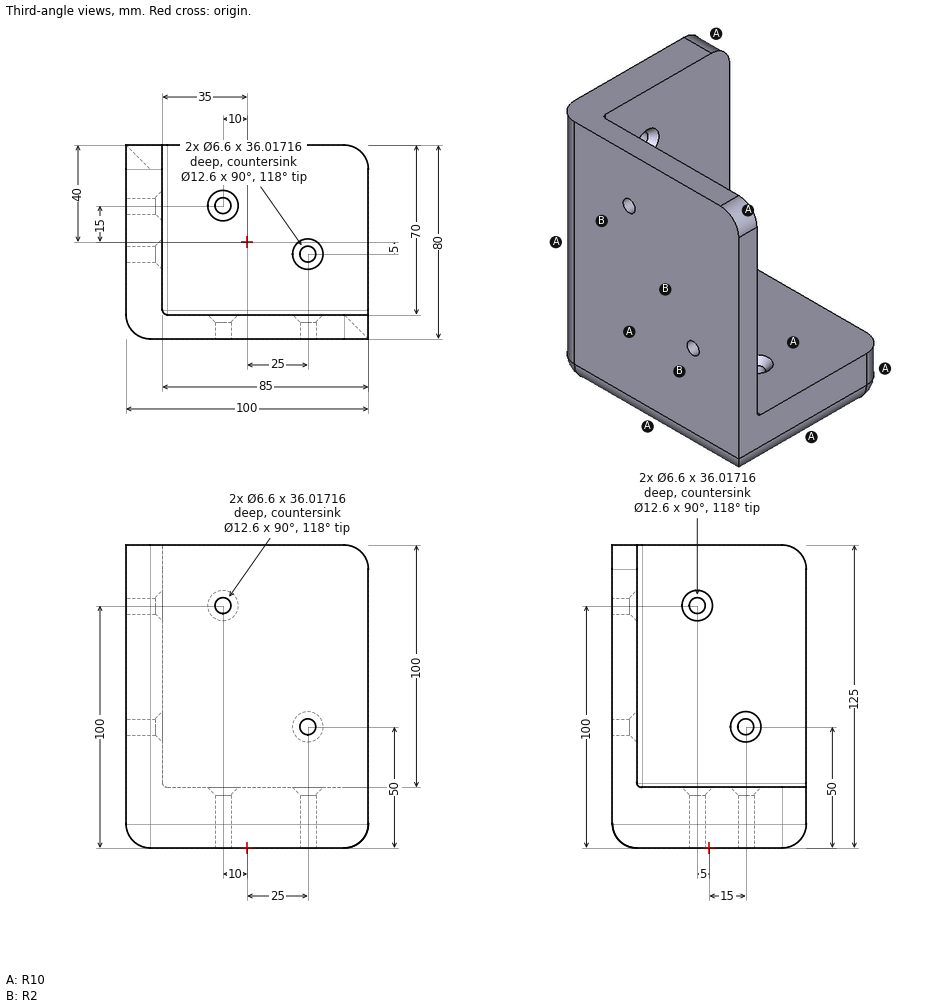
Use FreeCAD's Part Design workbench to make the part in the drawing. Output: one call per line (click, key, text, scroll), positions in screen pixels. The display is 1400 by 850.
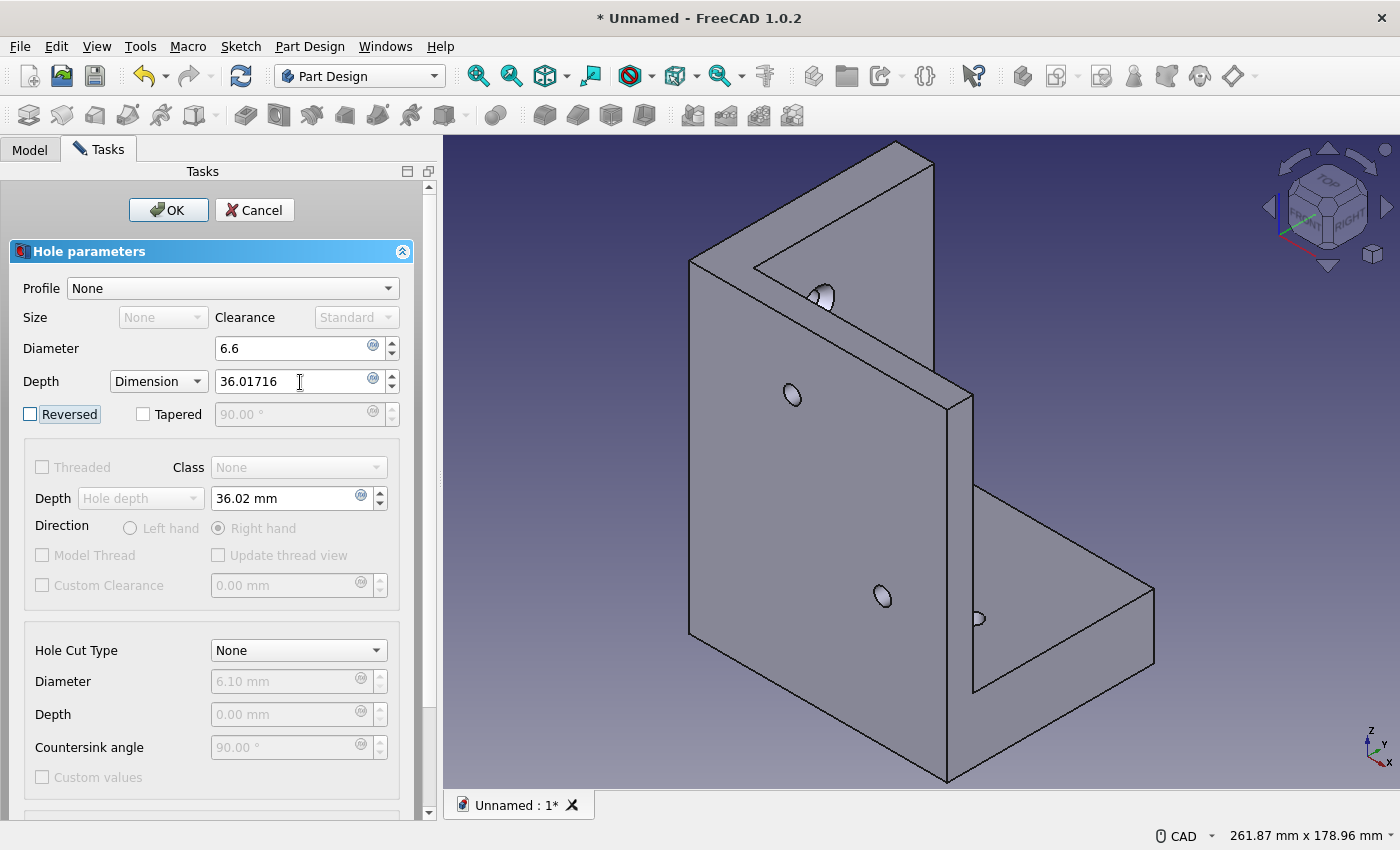
click(300, 650)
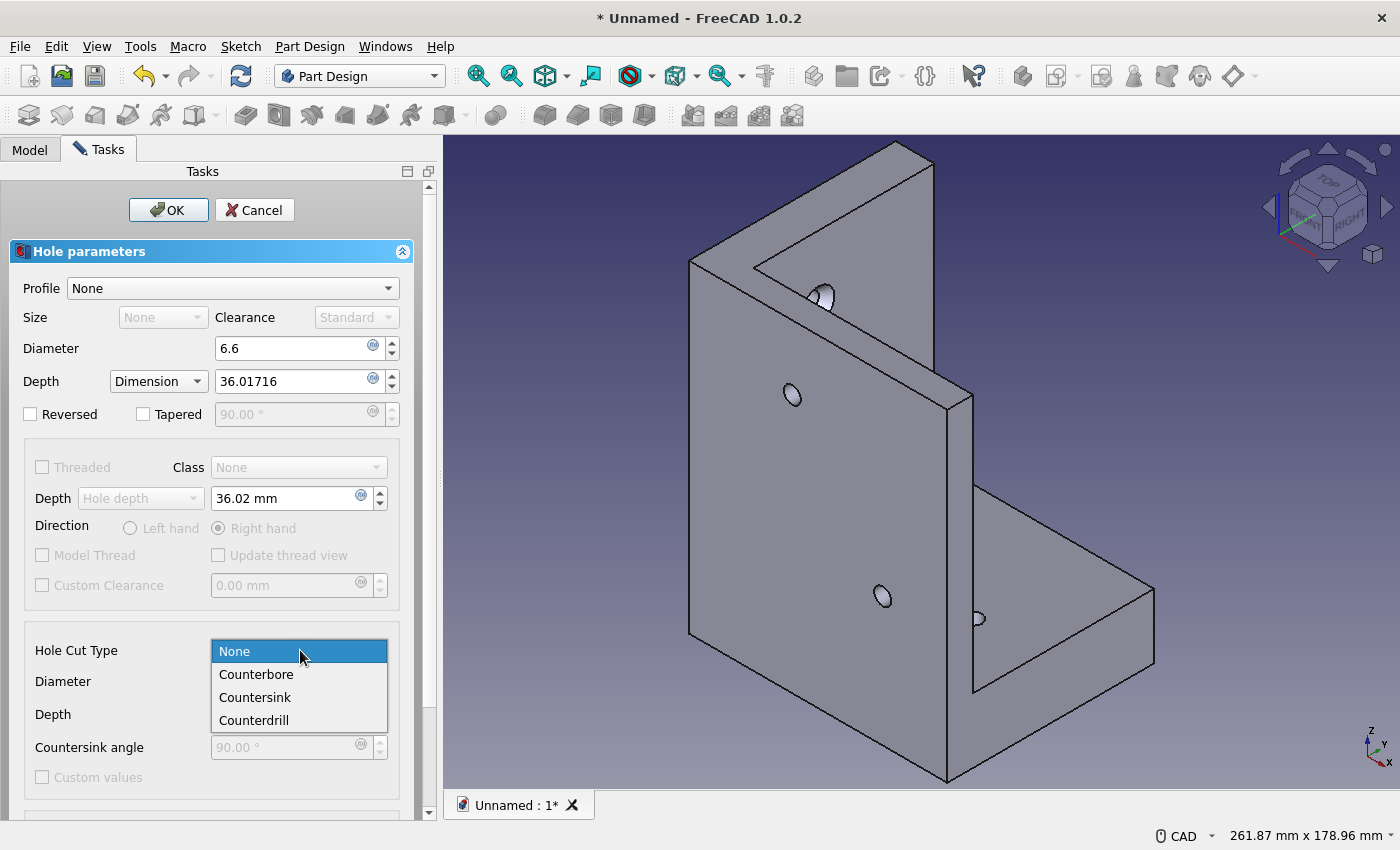
click(298, 698)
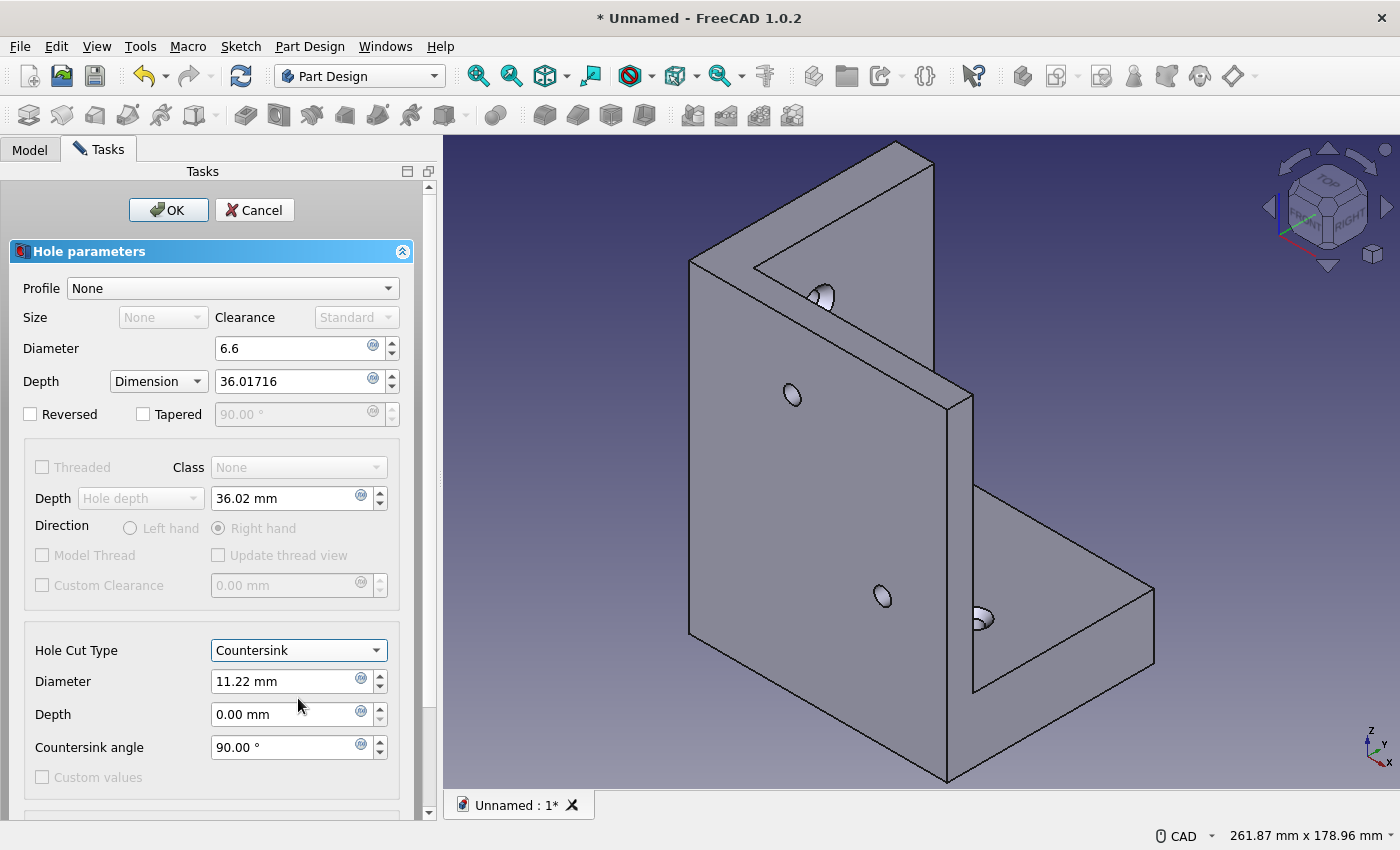
triple_click(292, 682)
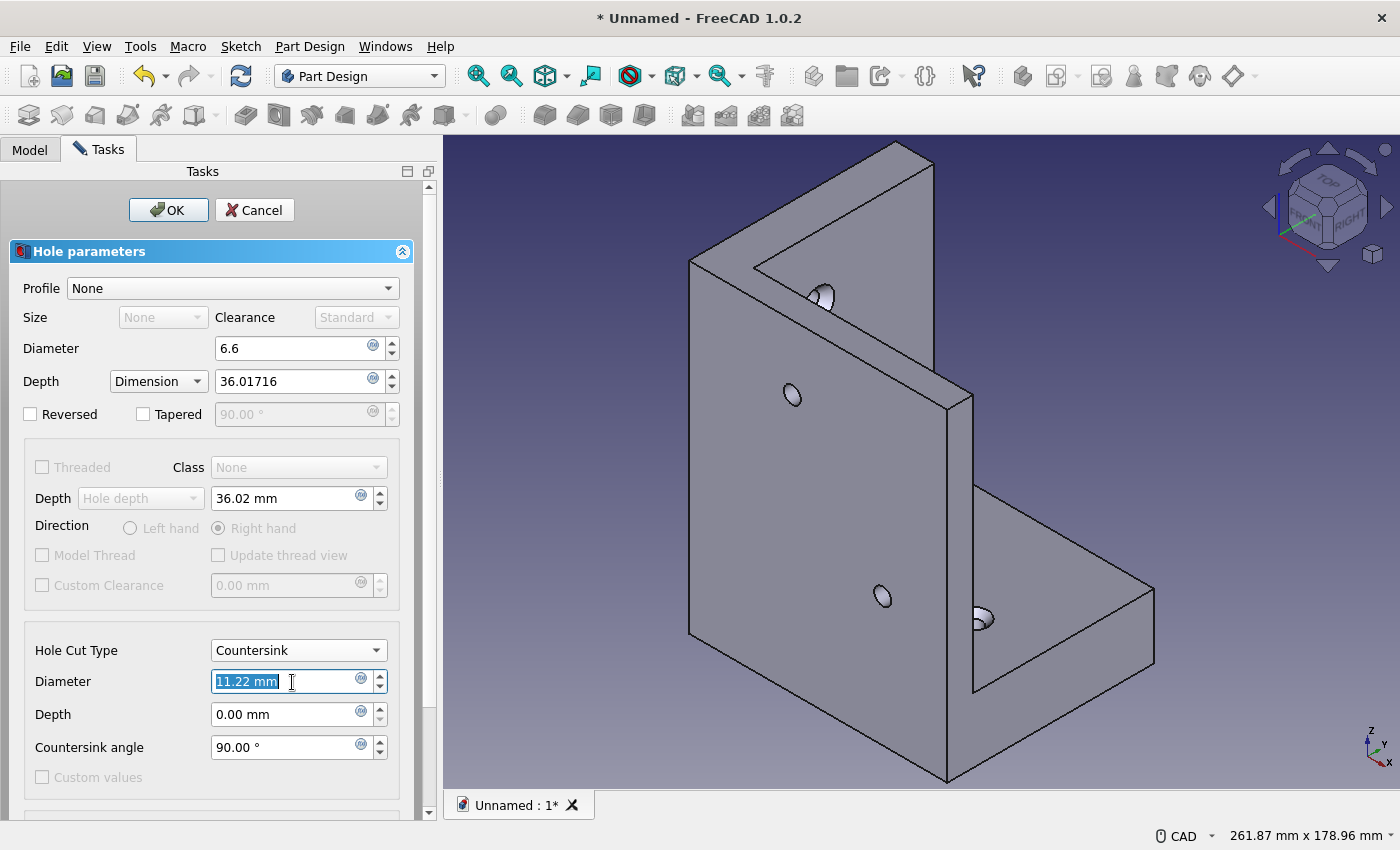
text(12.6)
key(Tab)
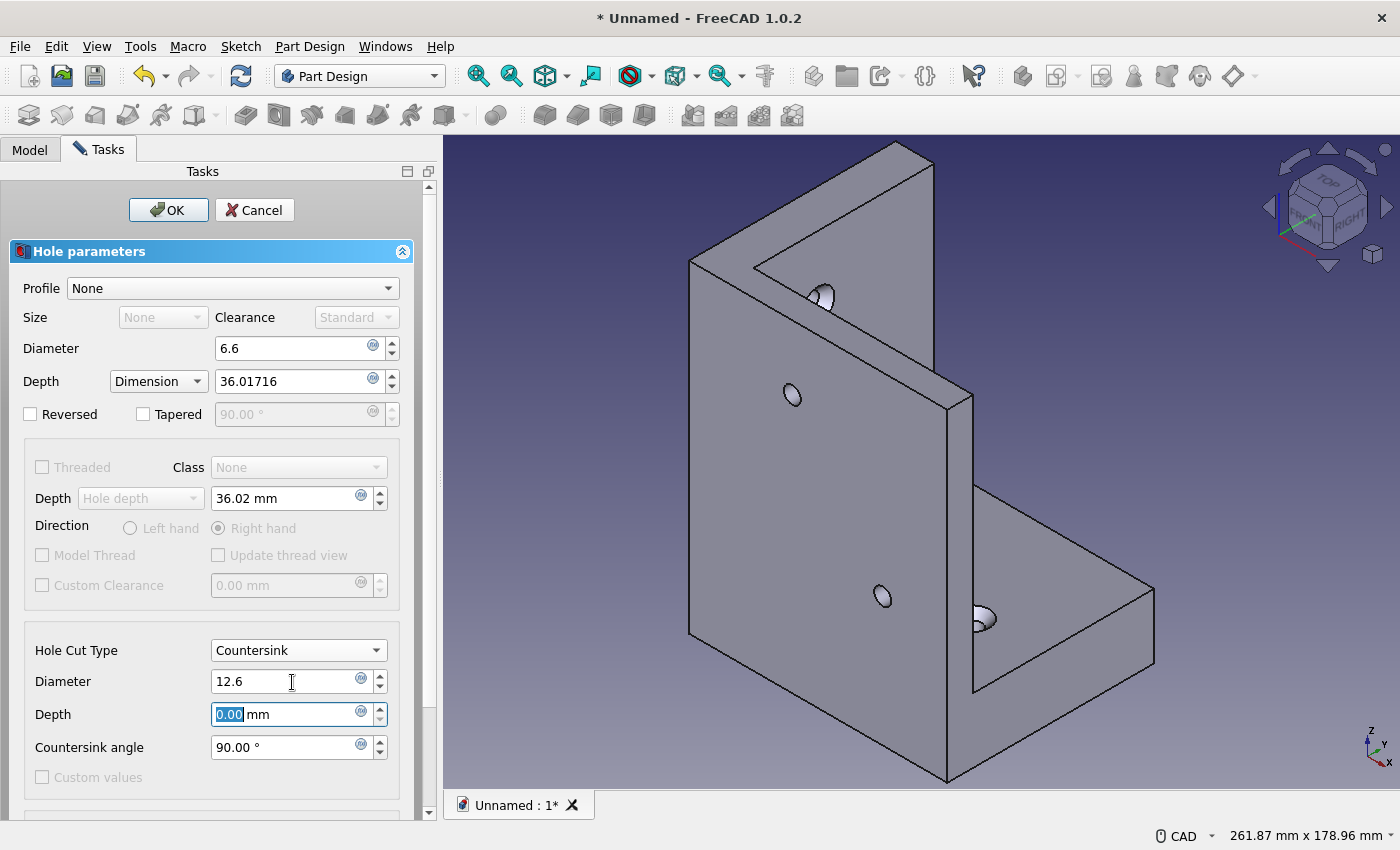
click(169, 210)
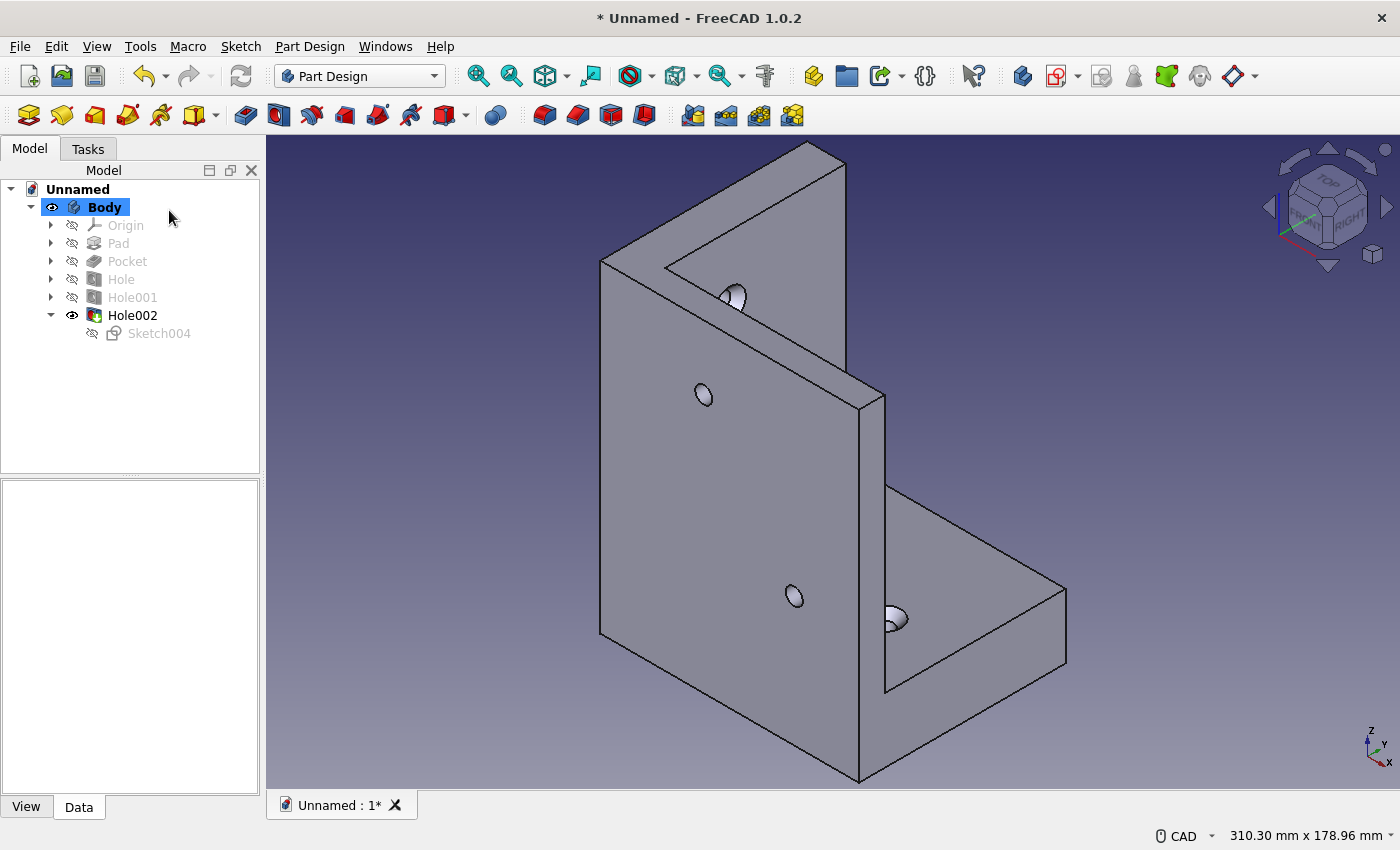
click(872, 401)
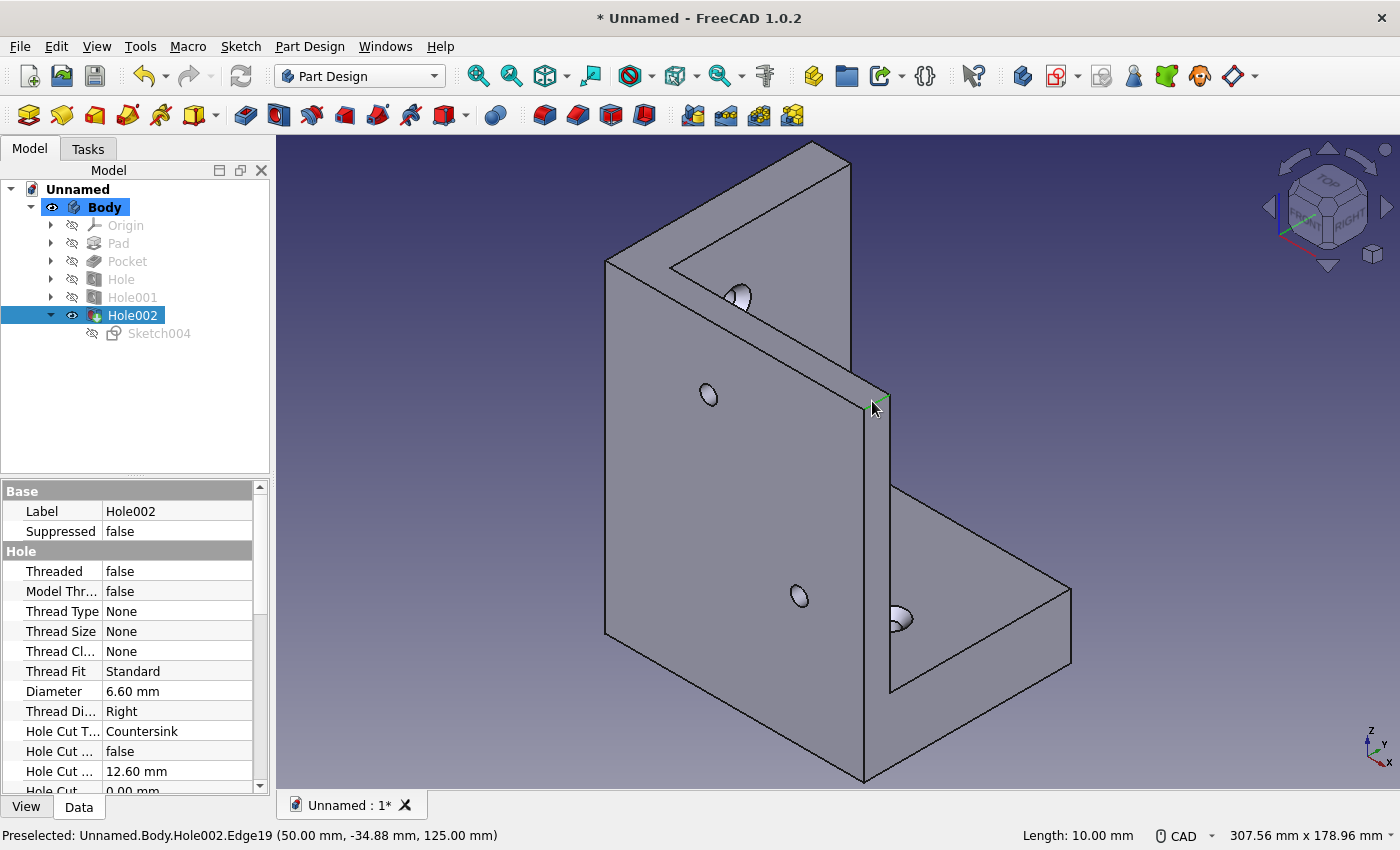
key(2)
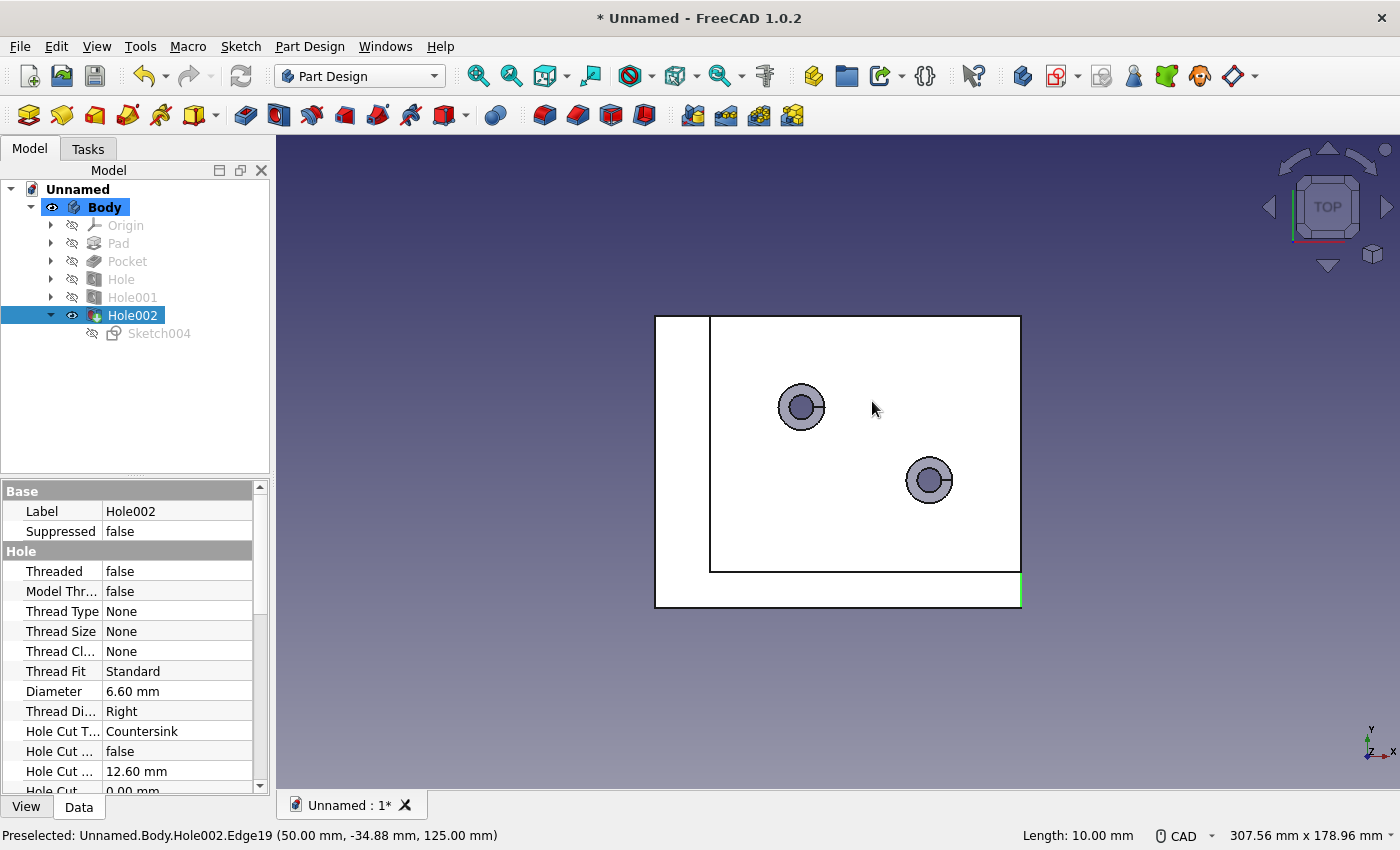
click(479, 76)